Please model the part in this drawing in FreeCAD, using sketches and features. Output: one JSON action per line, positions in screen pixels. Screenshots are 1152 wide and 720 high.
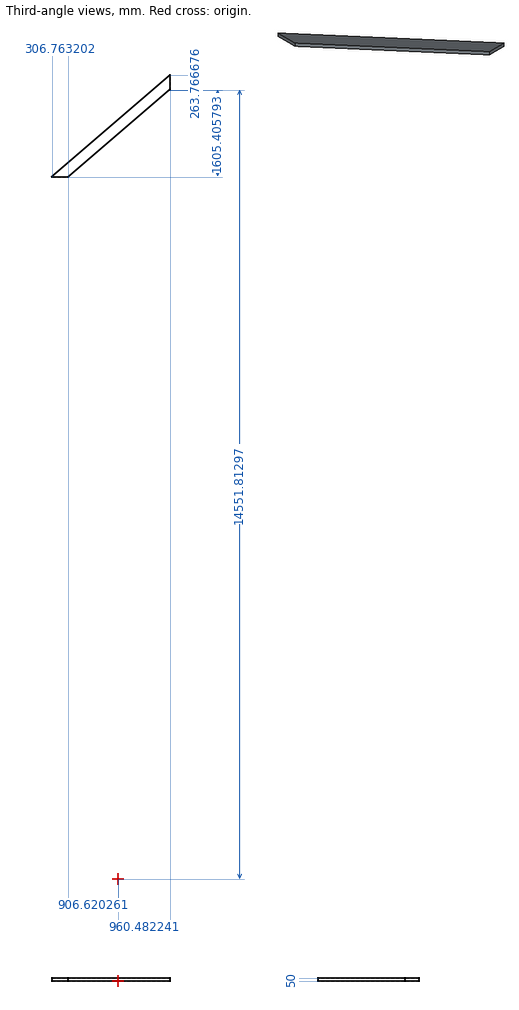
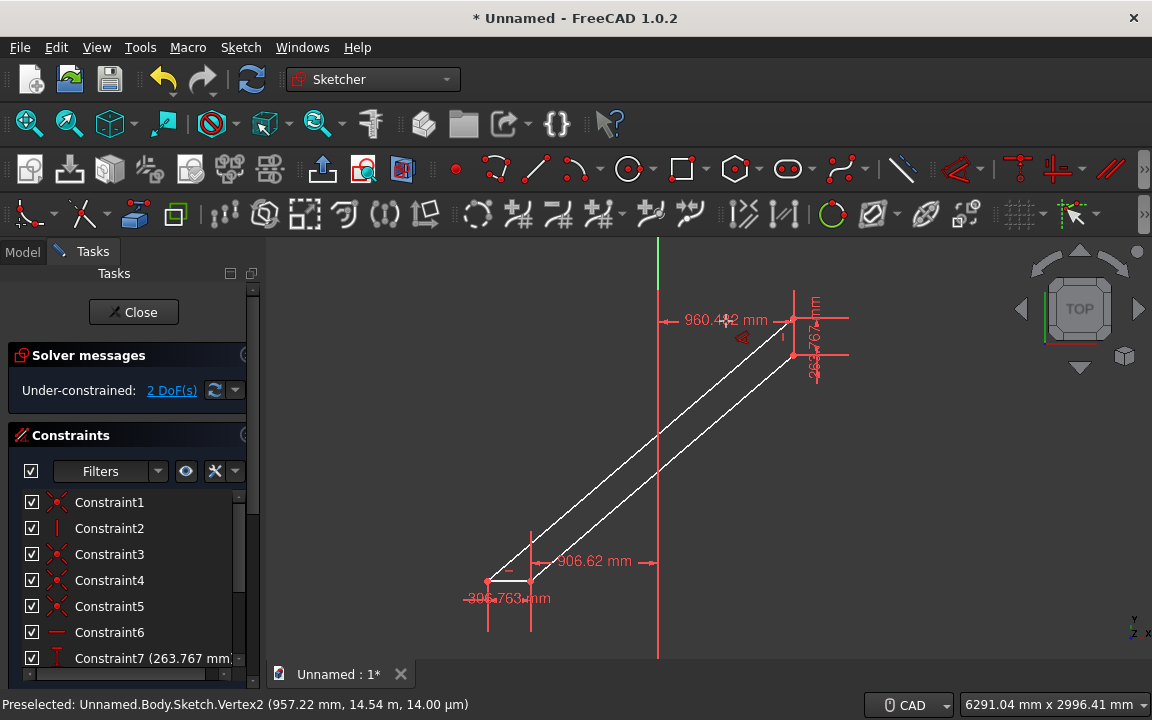
{"action": "left_click", "coordinate": [794, 355]}
{"action": "left_click", "coordinate": [828, 493]}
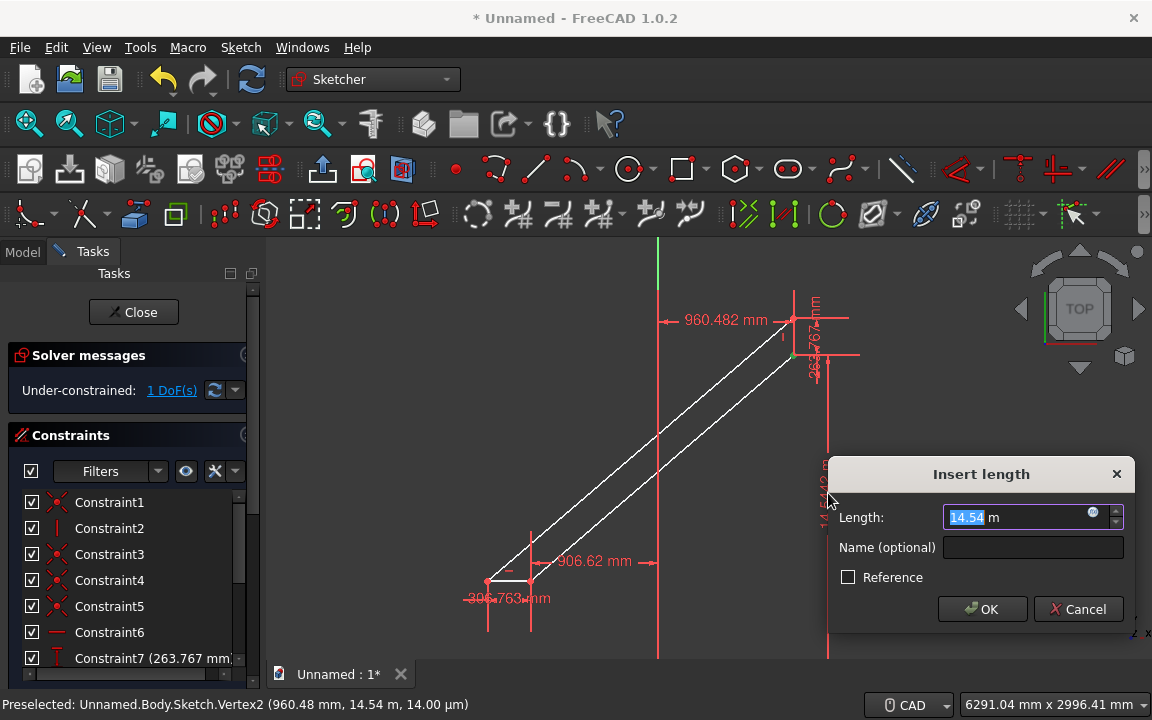
{"action": "key", "text": "ctrl+a"}
{"action": "type", "text": "14551.81297 mm"}
{"action": "key", "text": "Return"}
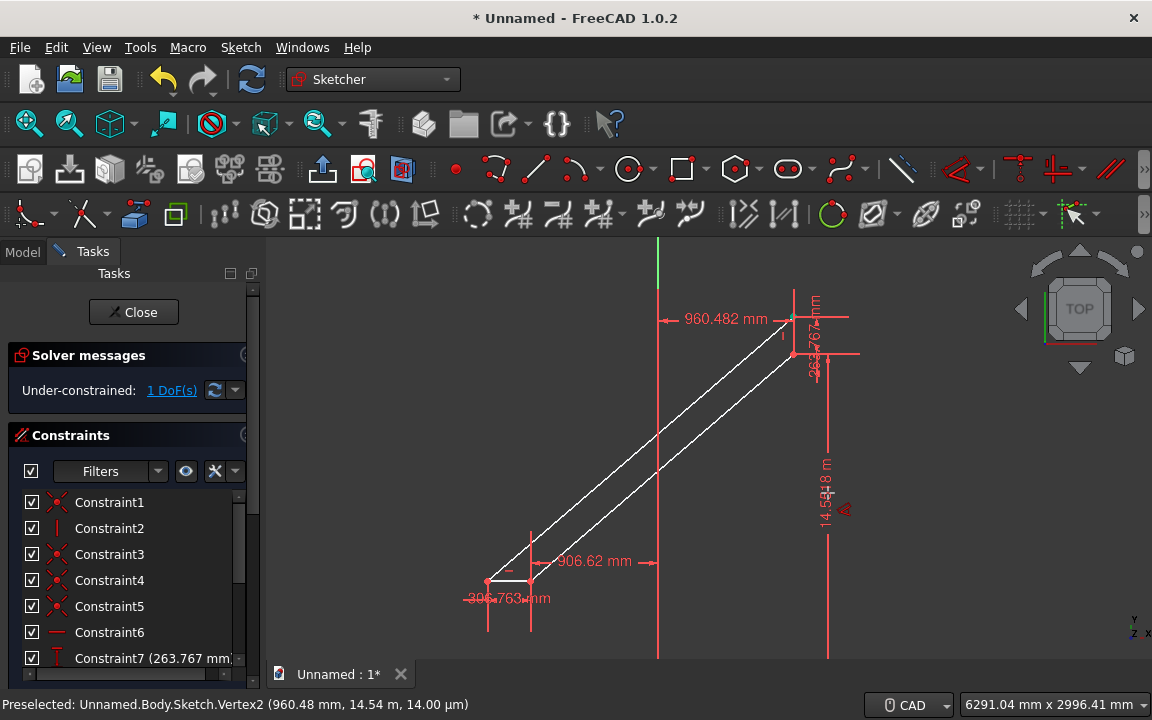
{"action": "left_click", "coordinate": [610, 513]}
{"action": "left_click", "coordinate": [828, 468]}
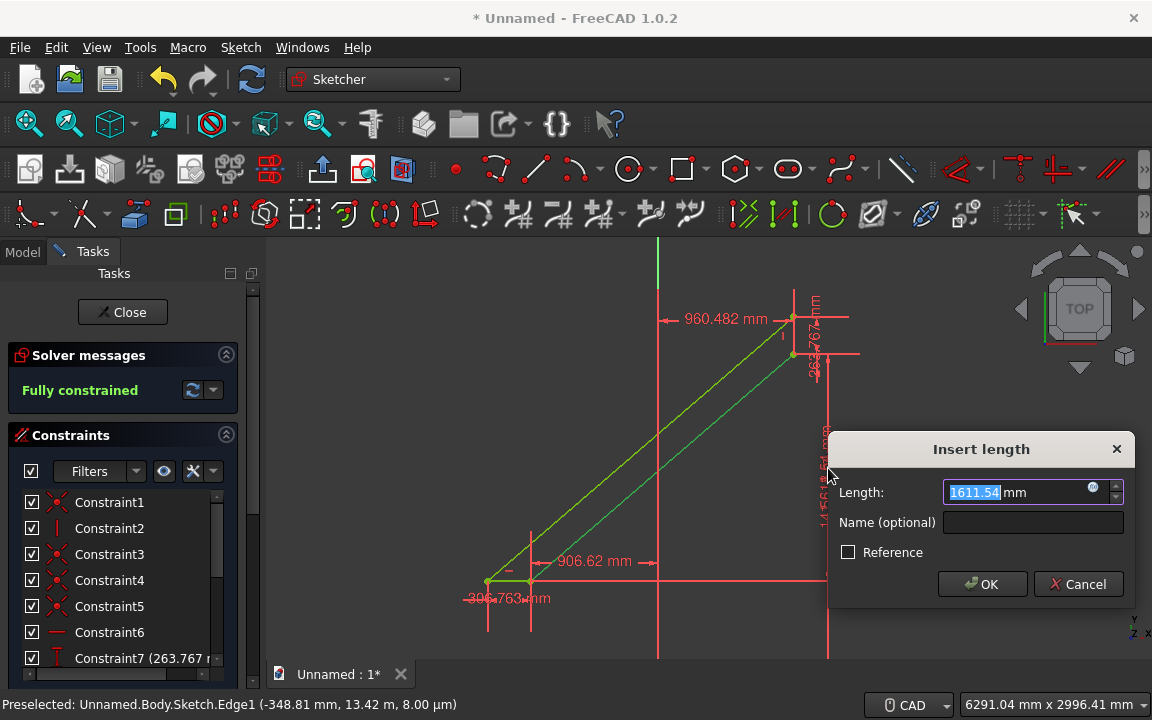
{"action": "type", "text": "1605.405793"}
{"action": "key", "text": "Return"}
{"action": "key", "text": "Escape"}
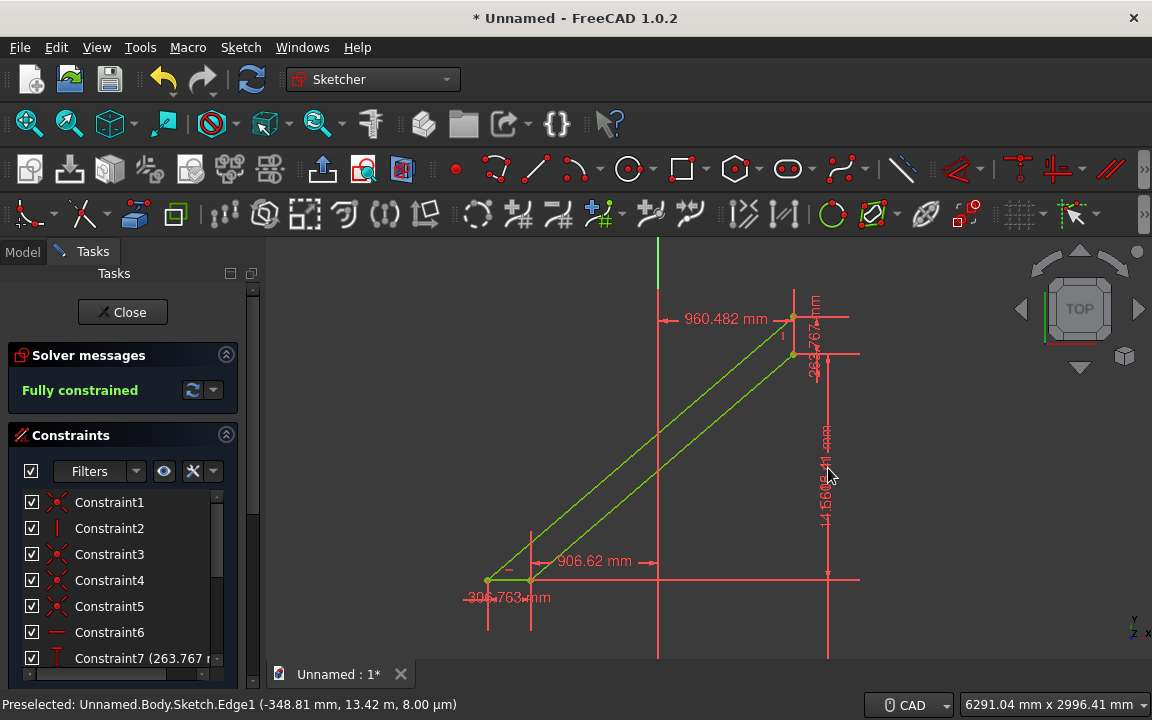
{"action": "left_click", "coordinate": [123, 312]}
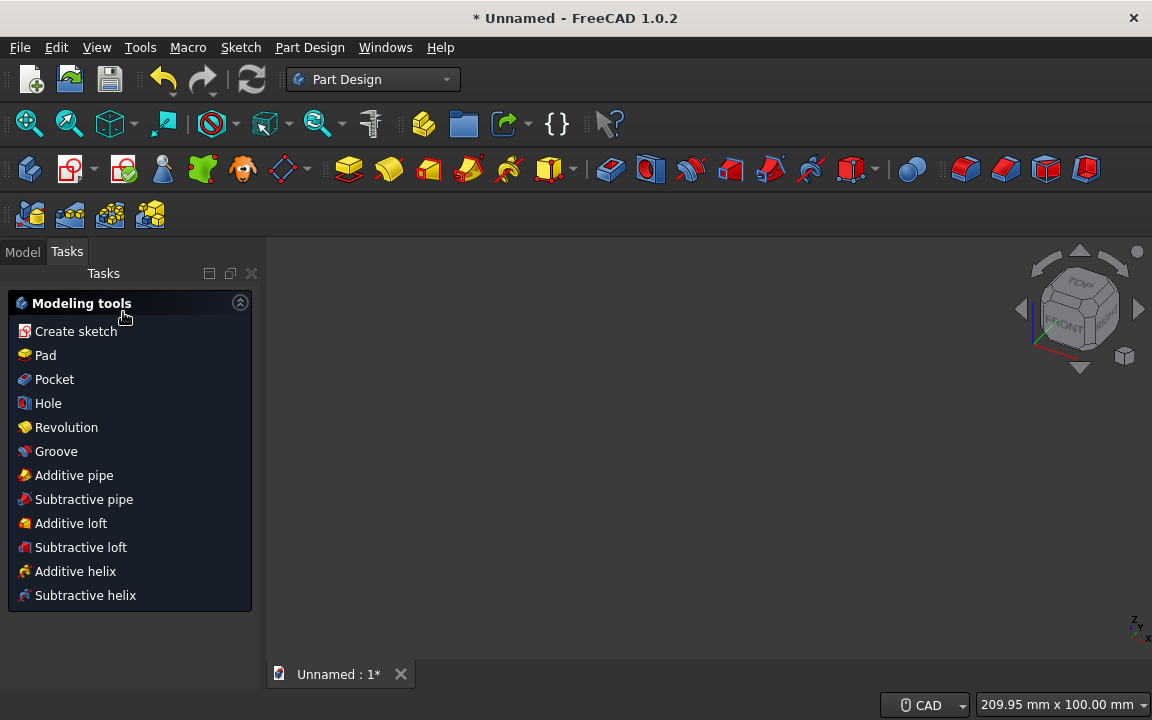
{"action": "left_click", "coordinate": [350, 170]}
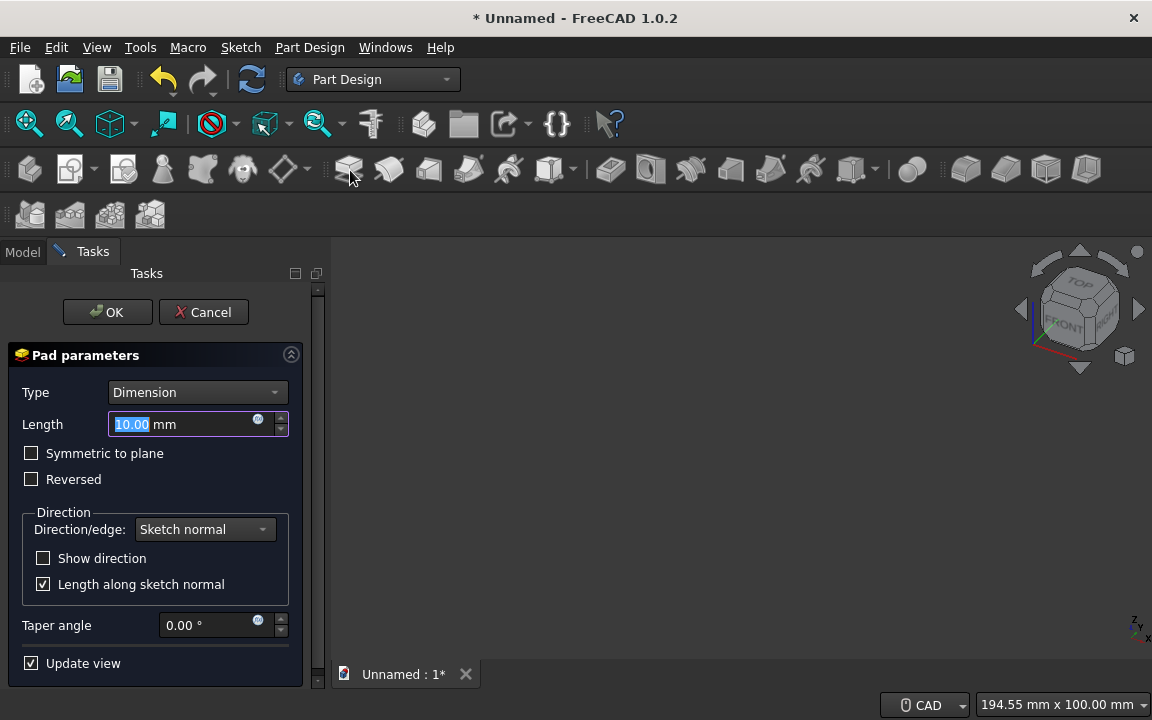
{"action": "type", "text": "50"}
{"action": "key", "text": "Tab"}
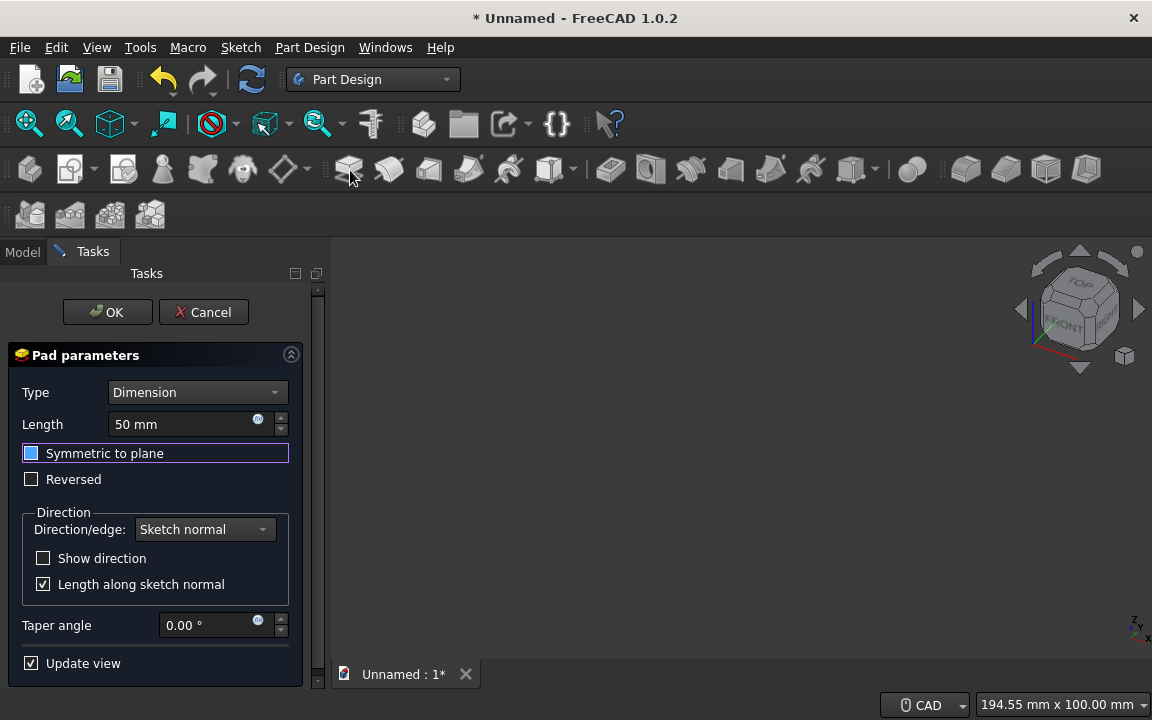
{"action": "left_click", "coordinate": [108, 312]}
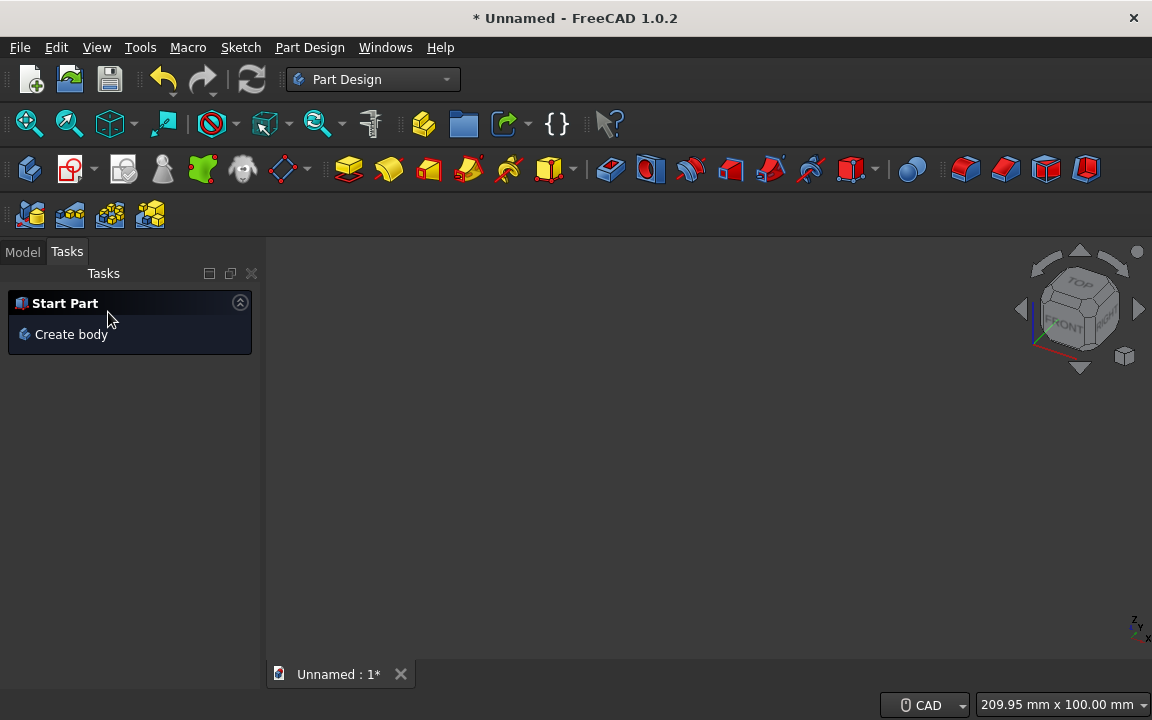
{"action": "key", "text": "0"}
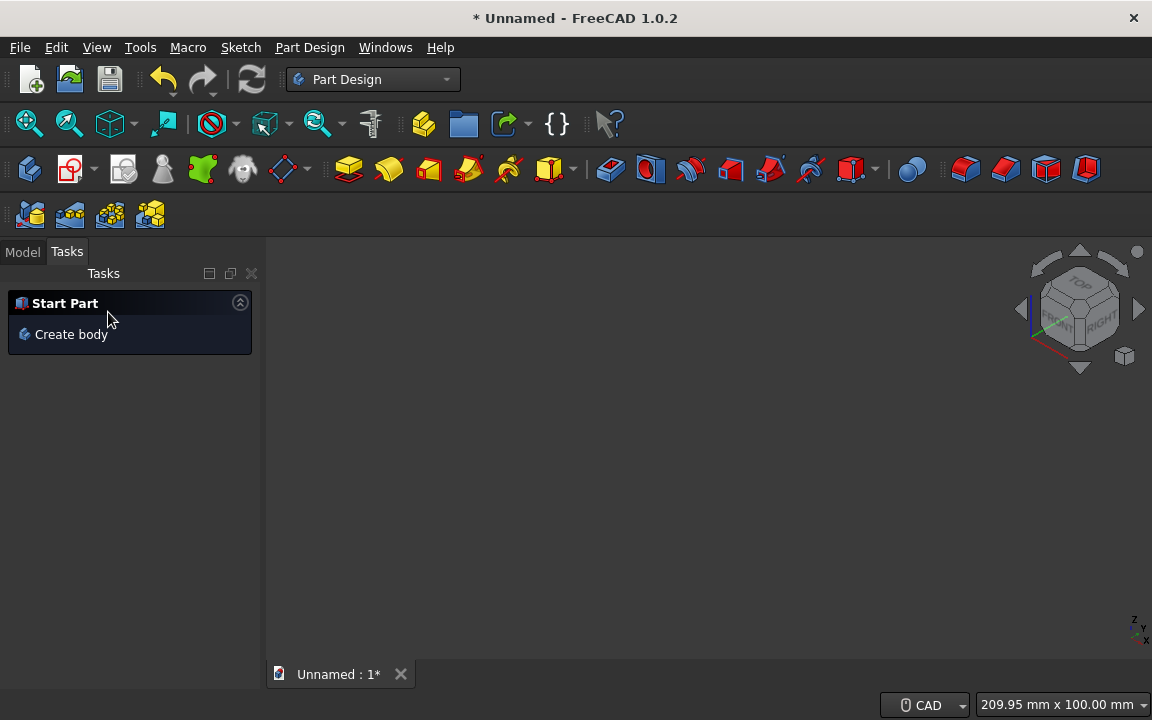
{"action": "key", "text": "v f"}